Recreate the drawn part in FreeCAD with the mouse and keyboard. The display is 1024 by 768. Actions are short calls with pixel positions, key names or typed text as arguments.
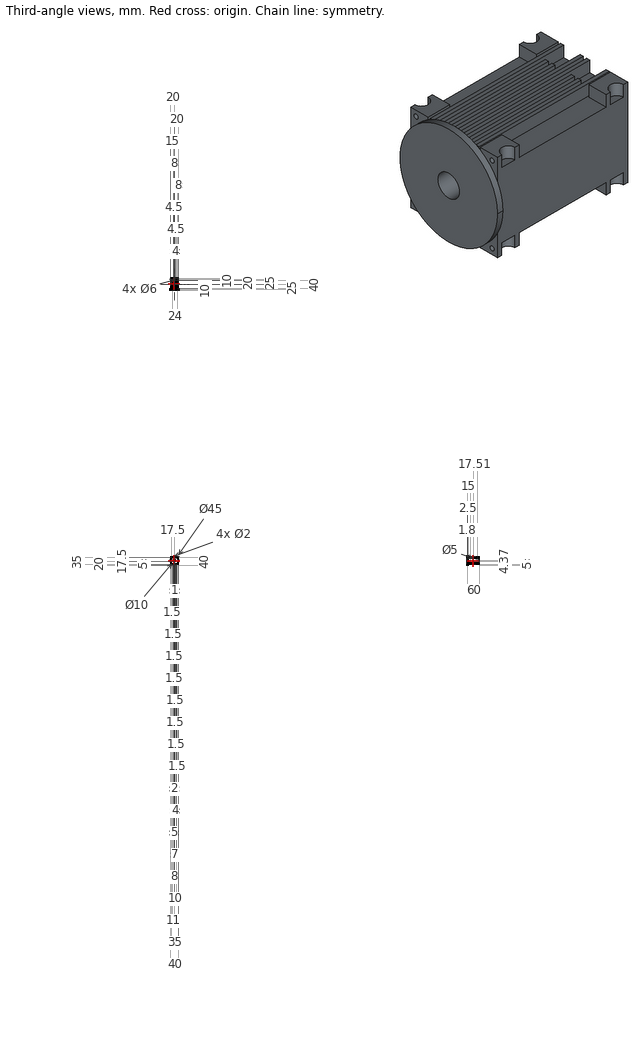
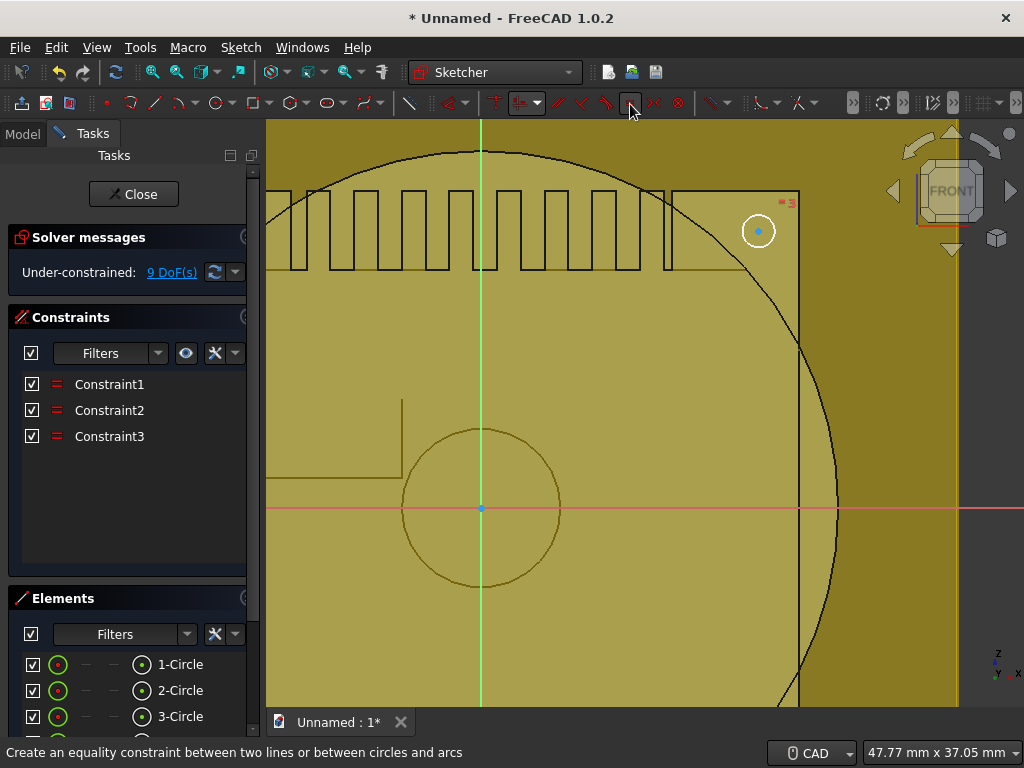
scroll(770, 220, down, 2)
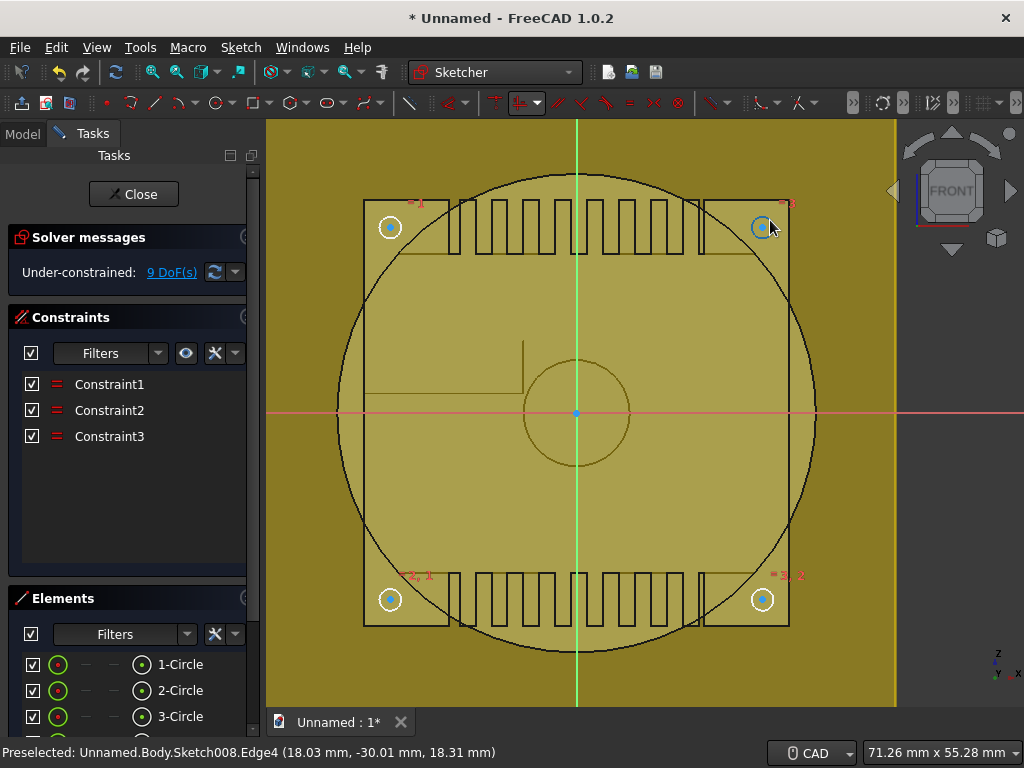
click(390, 228)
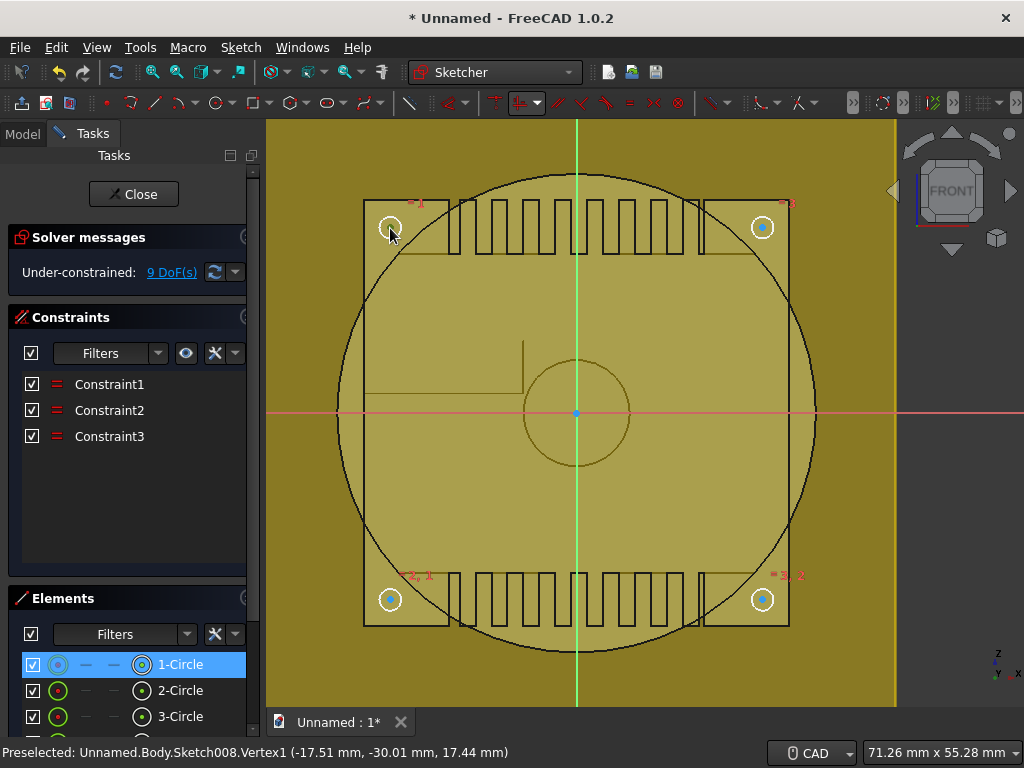
click(390, 600)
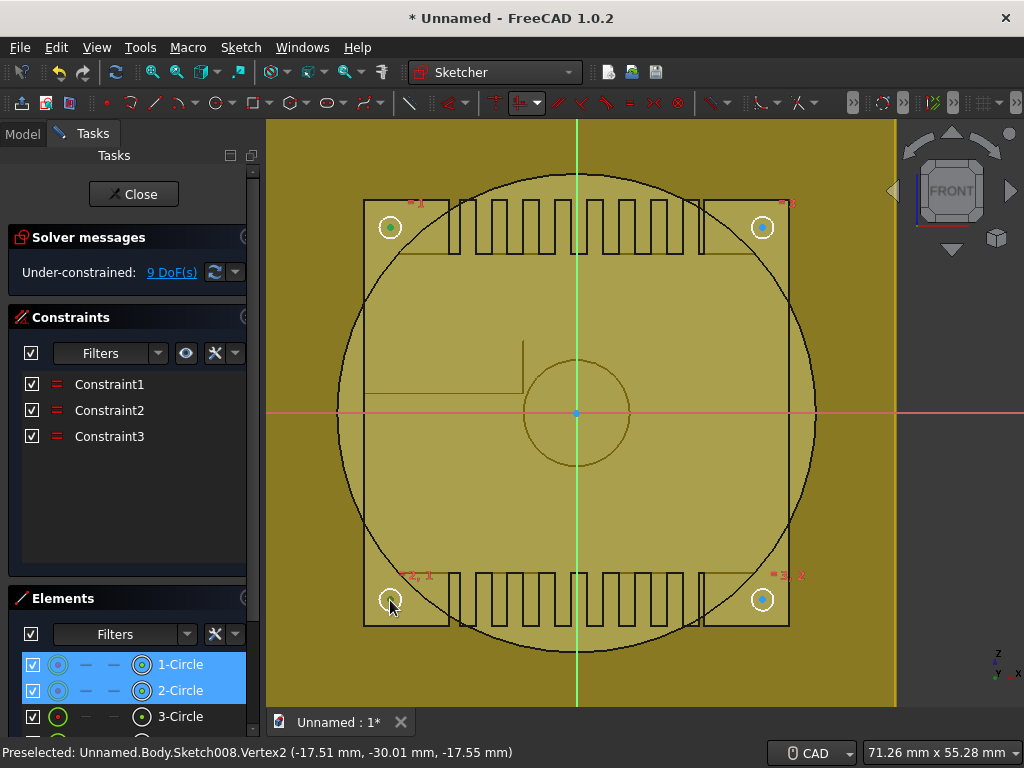
click(540, 104)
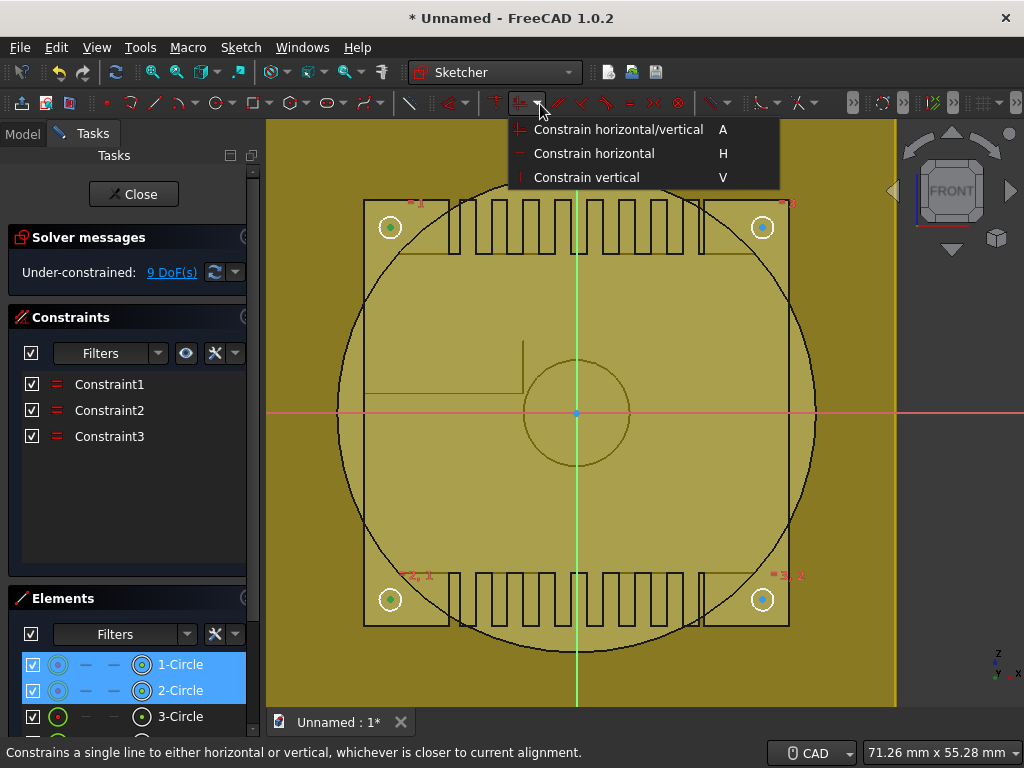
click(644, 177)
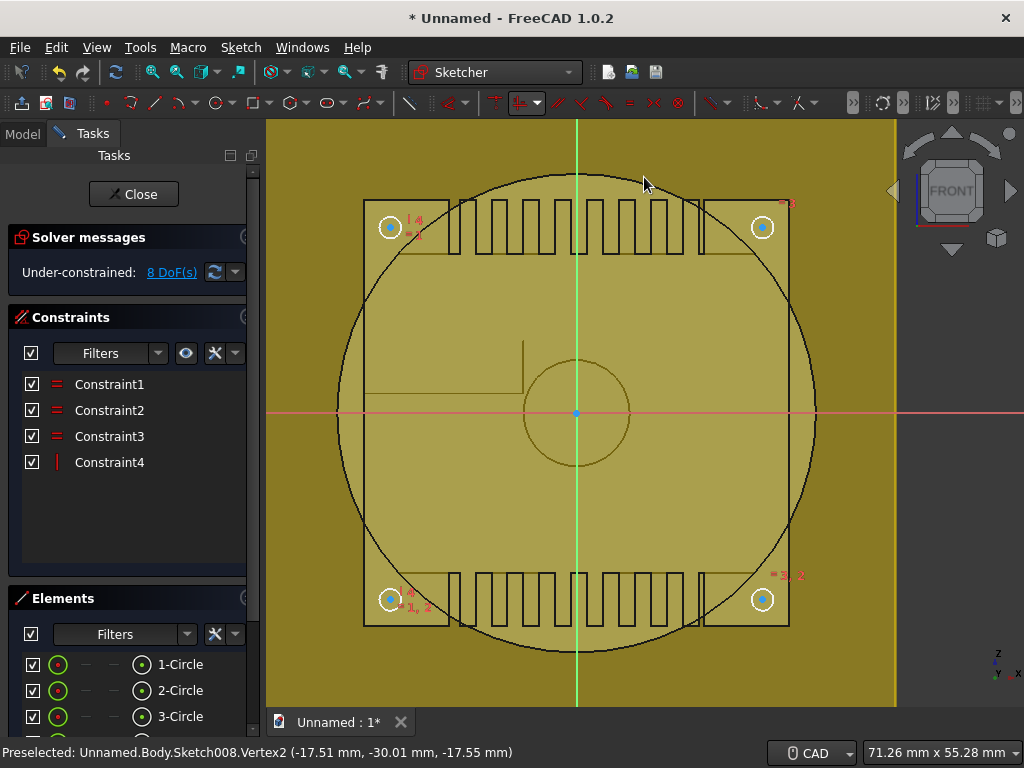
click(390, 600)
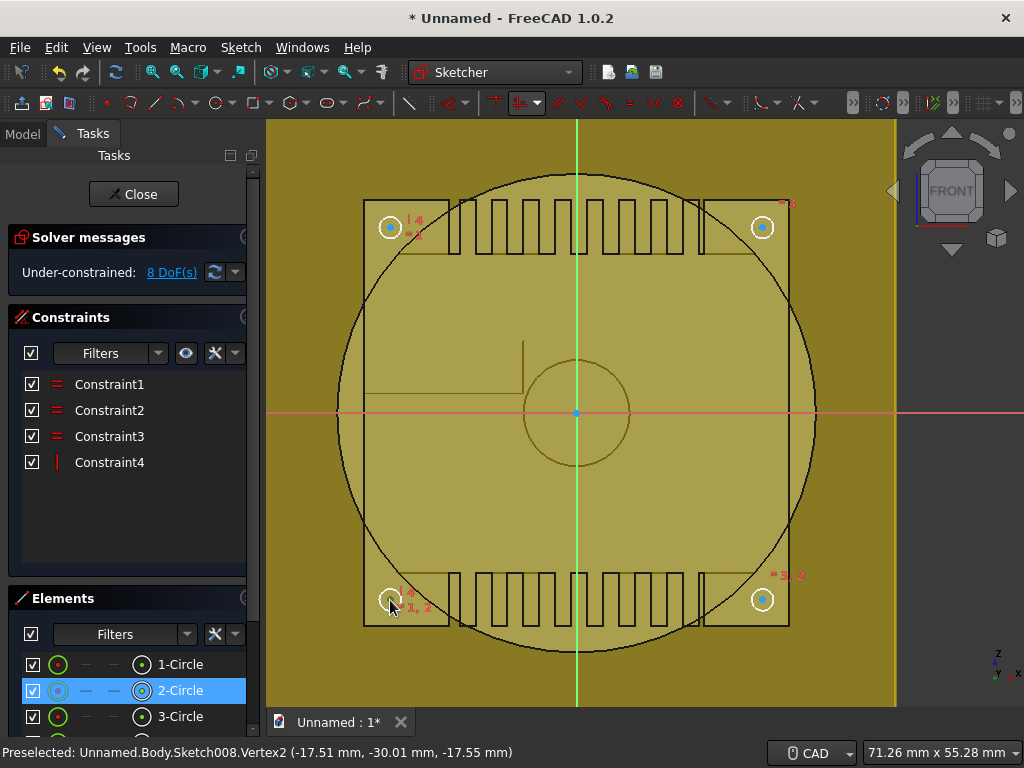
click(763, 600)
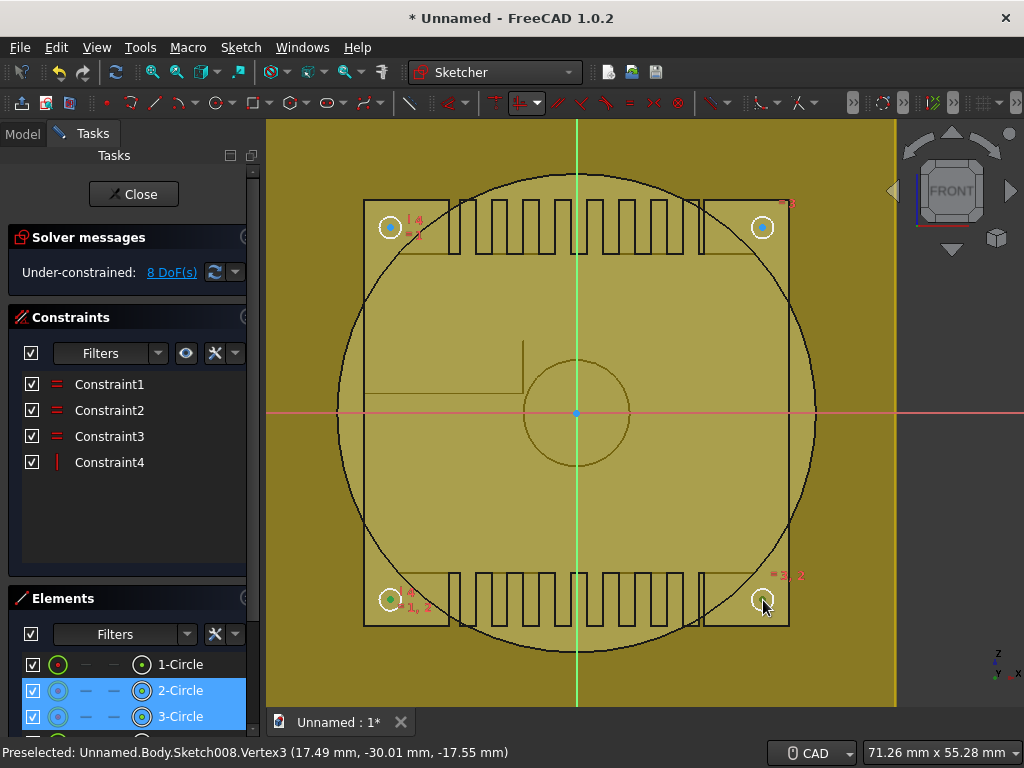
click(540, 104)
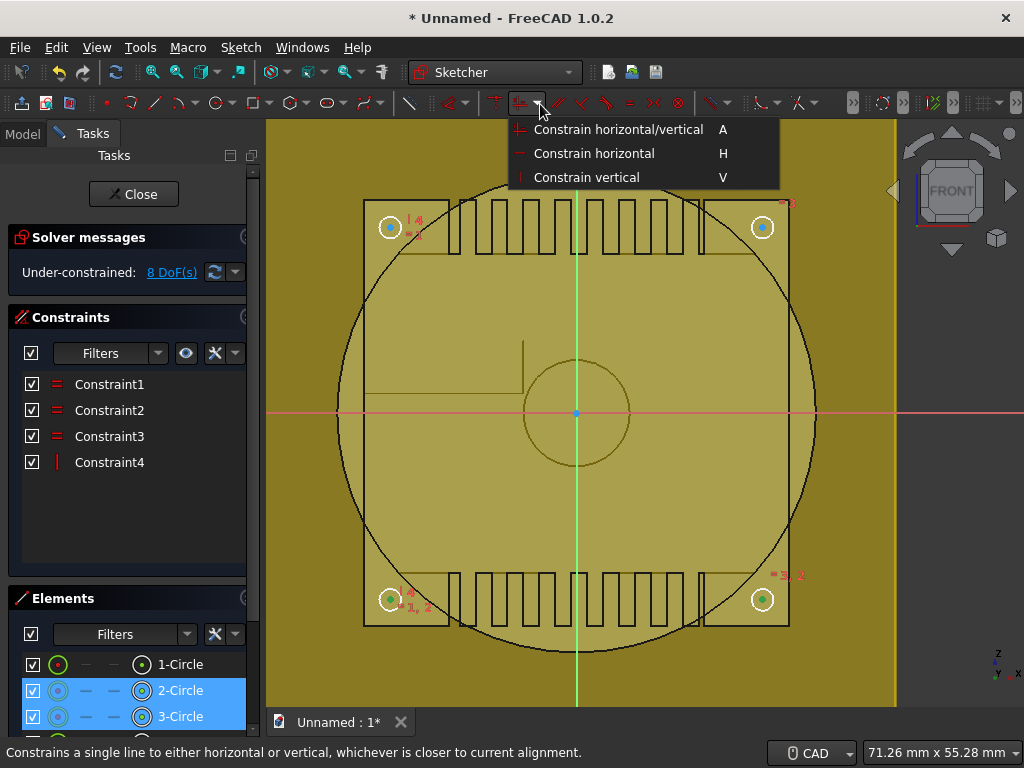
click(644, 153)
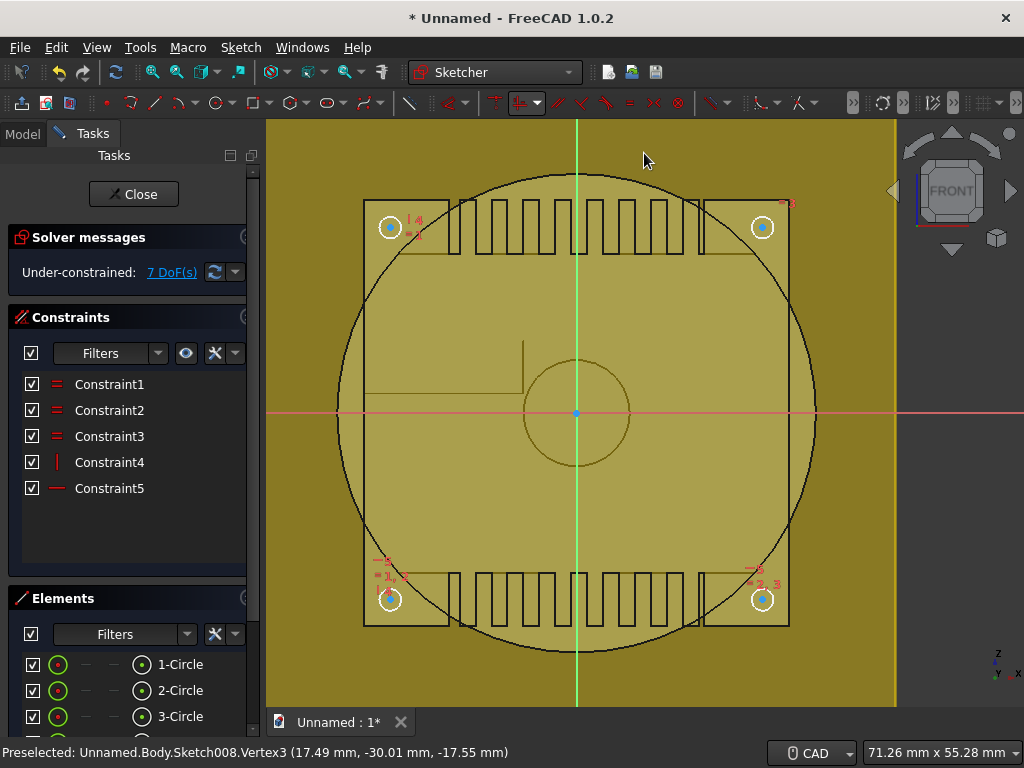
click(763, 600)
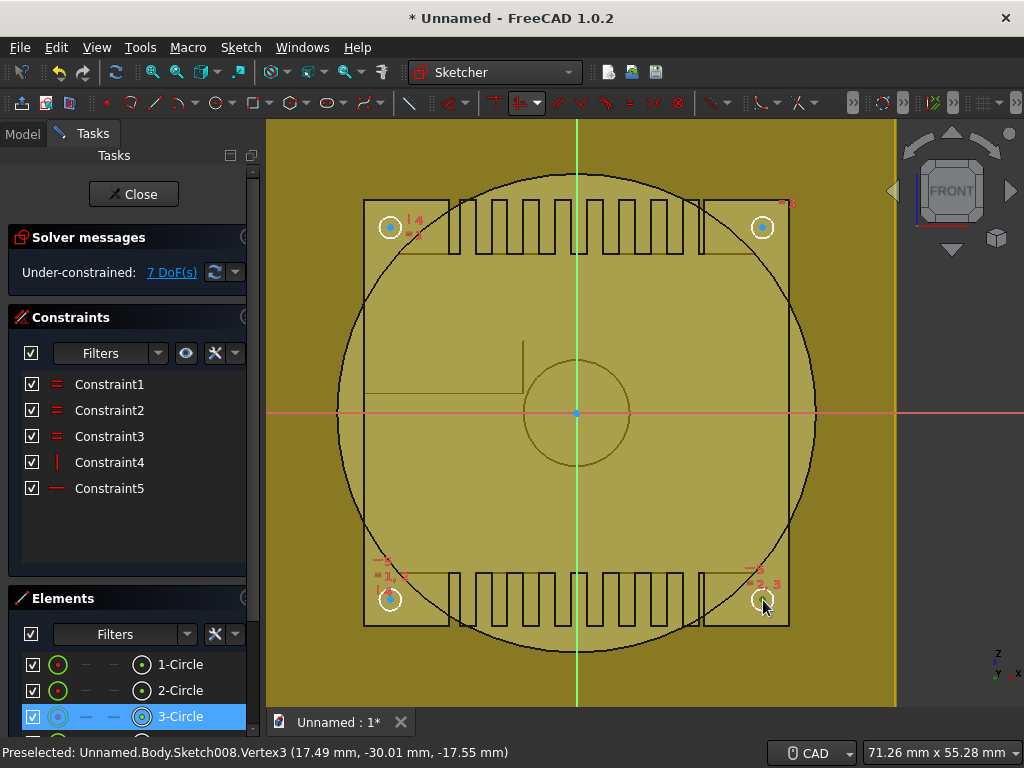
click(763, 228)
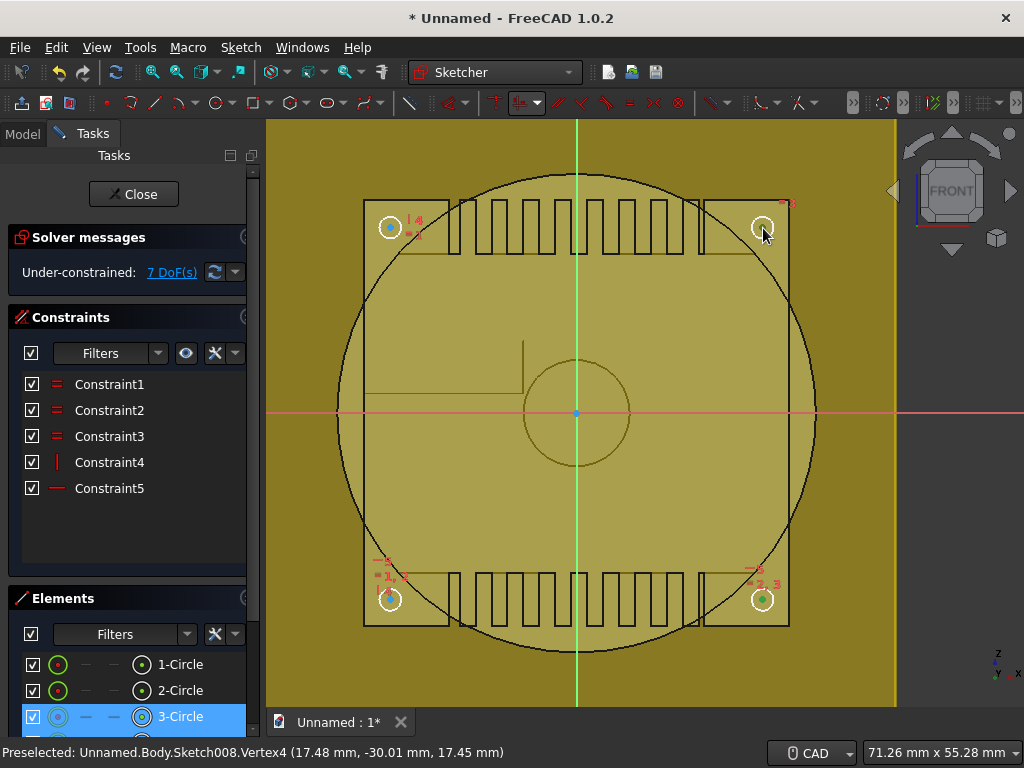
key(v)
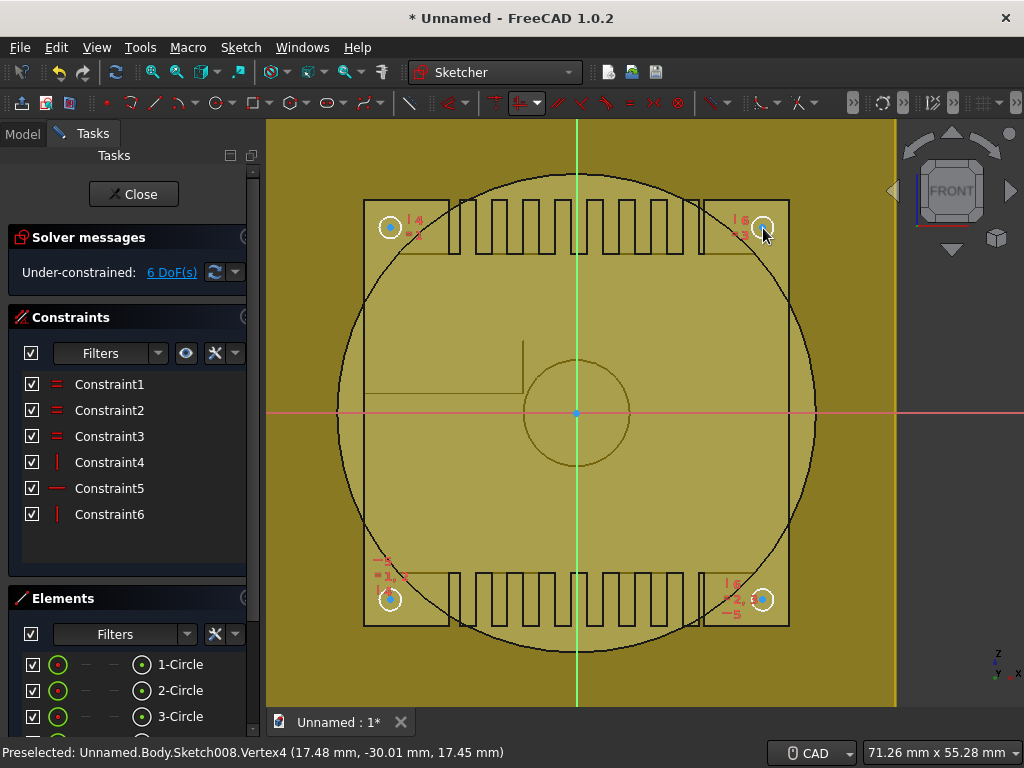
click(390, 228)